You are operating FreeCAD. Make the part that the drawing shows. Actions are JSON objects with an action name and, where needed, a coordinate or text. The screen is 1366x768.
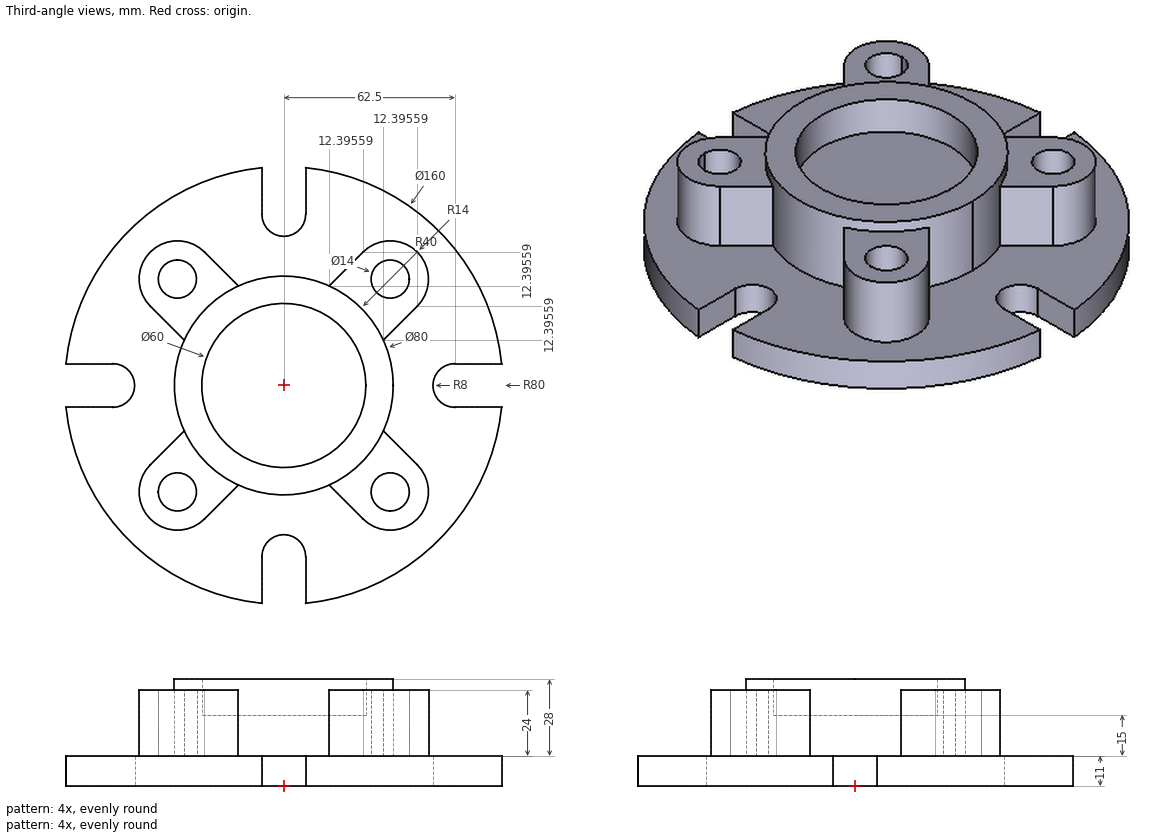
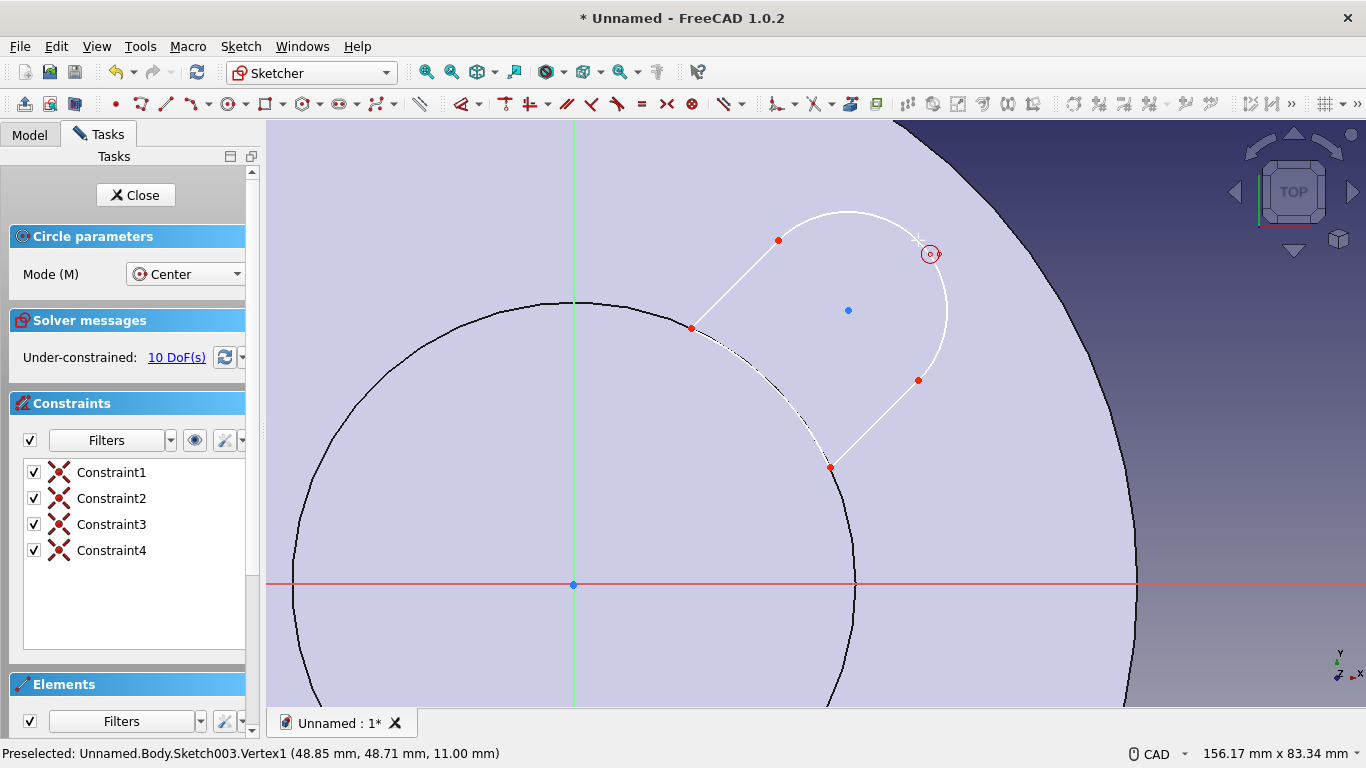
{"action": "left_click", "coordinate": [848, 310]}
{"action": "left_click", "coordinate": [883, 275]}
{"action": "key", "text": "Escape"}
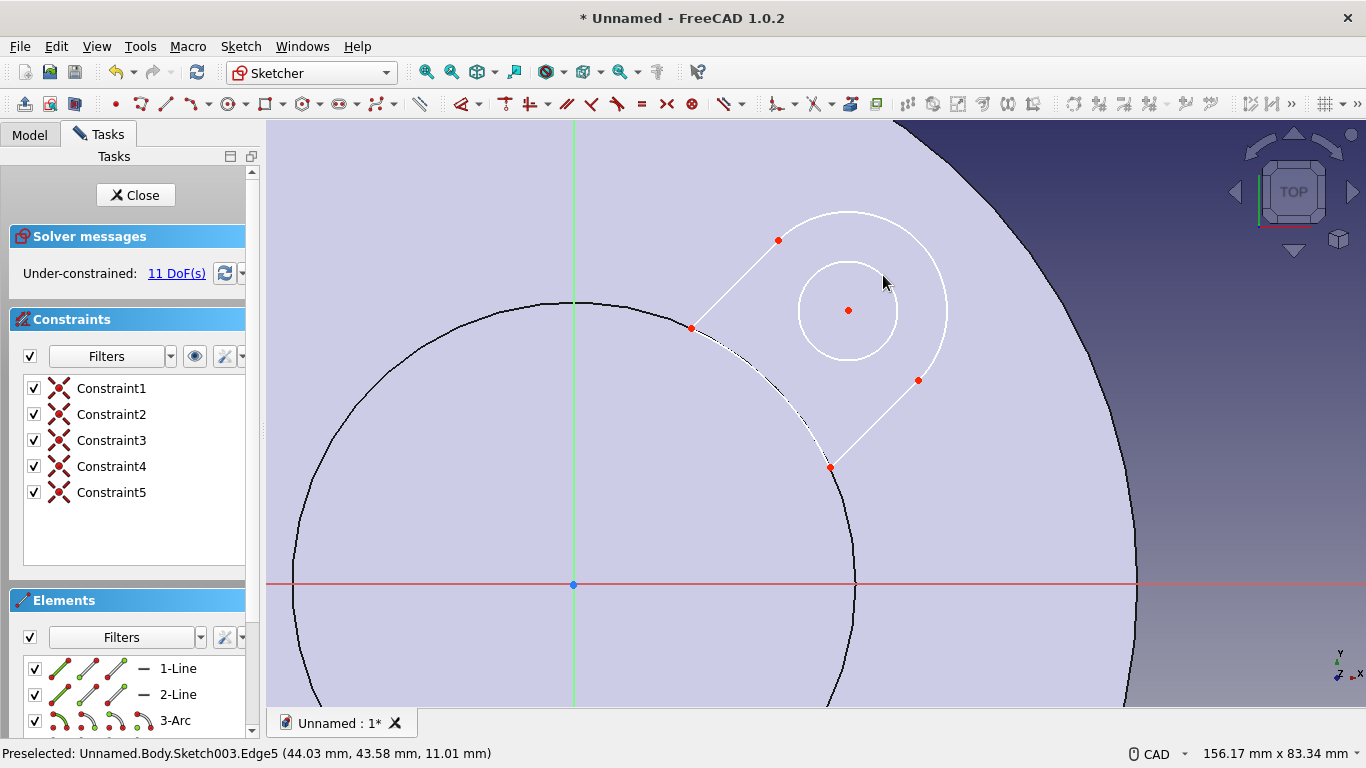
{"action": "left_click", "coordinate": [752, 267]}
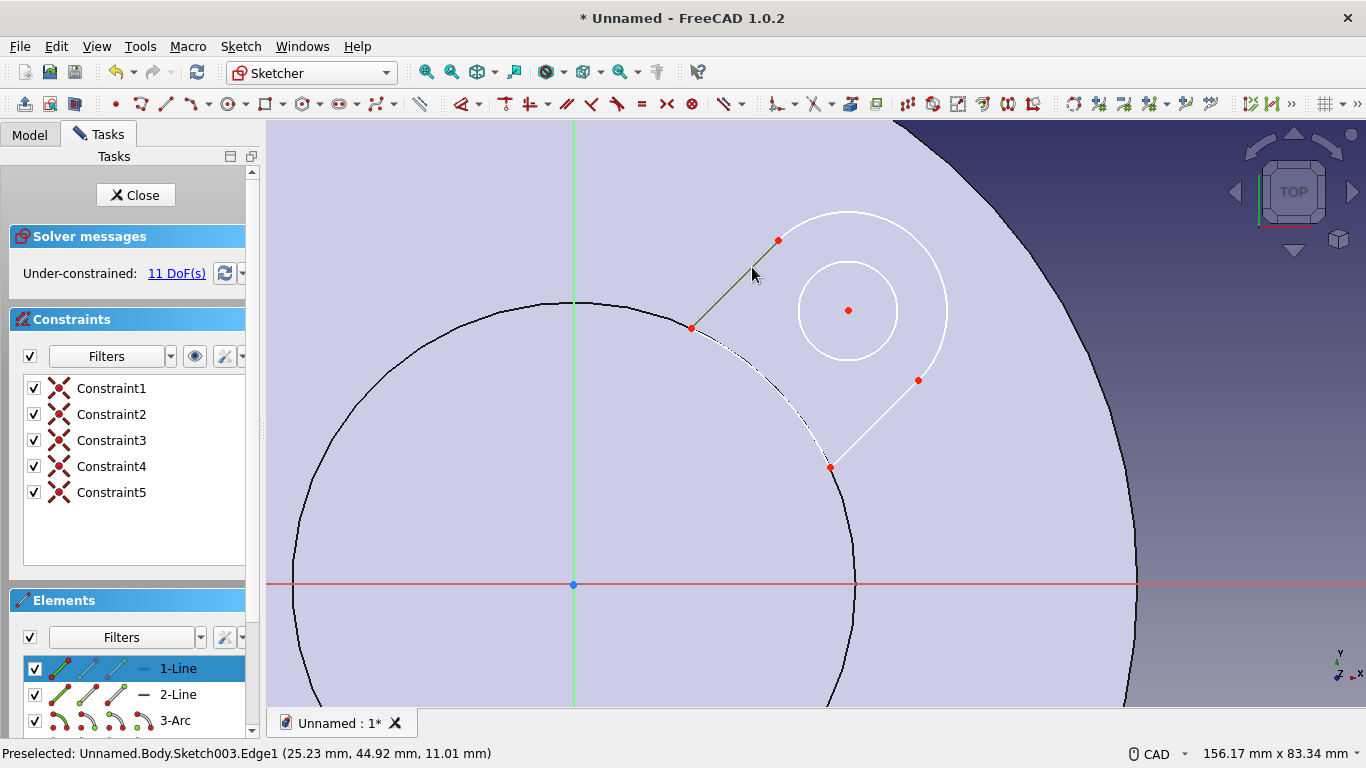
{"action": "left_click", "coordinate": [946, 296]}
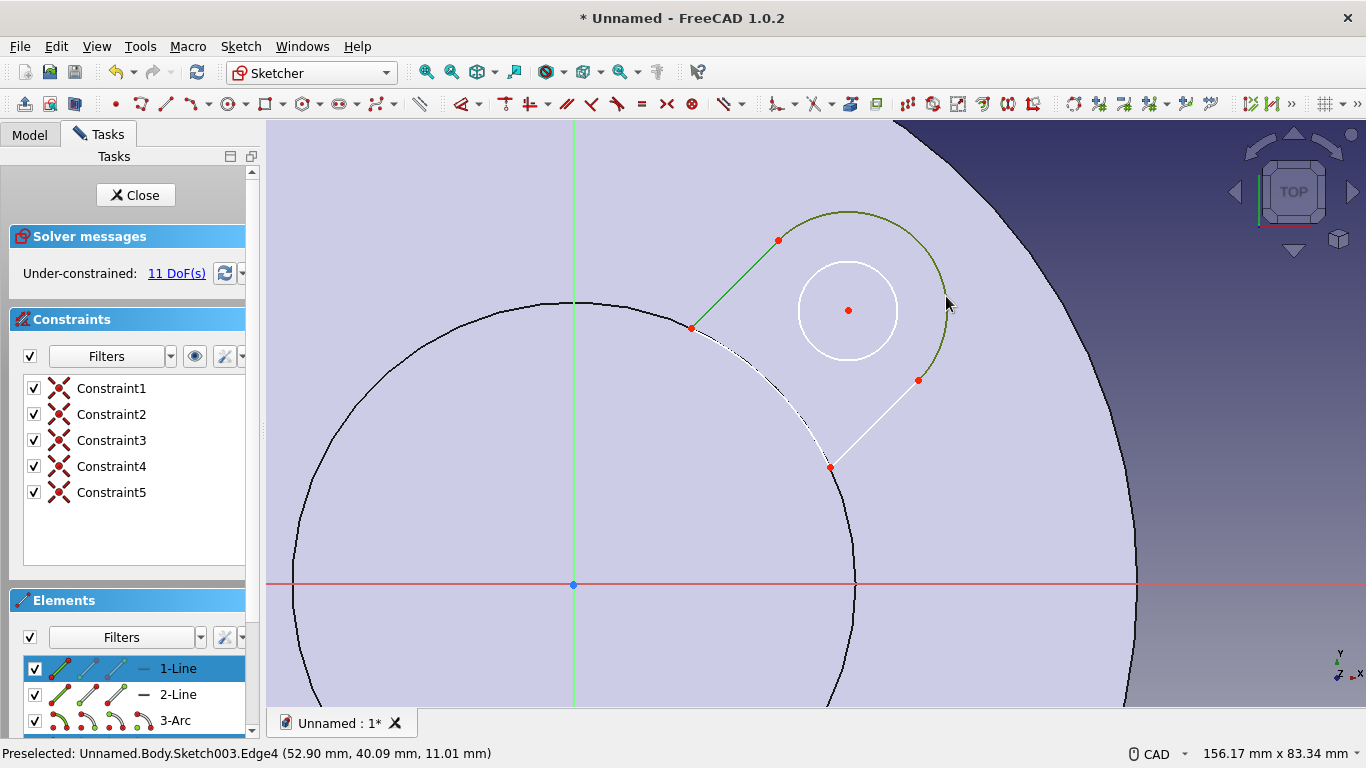
{"action": "key", "text": "t"}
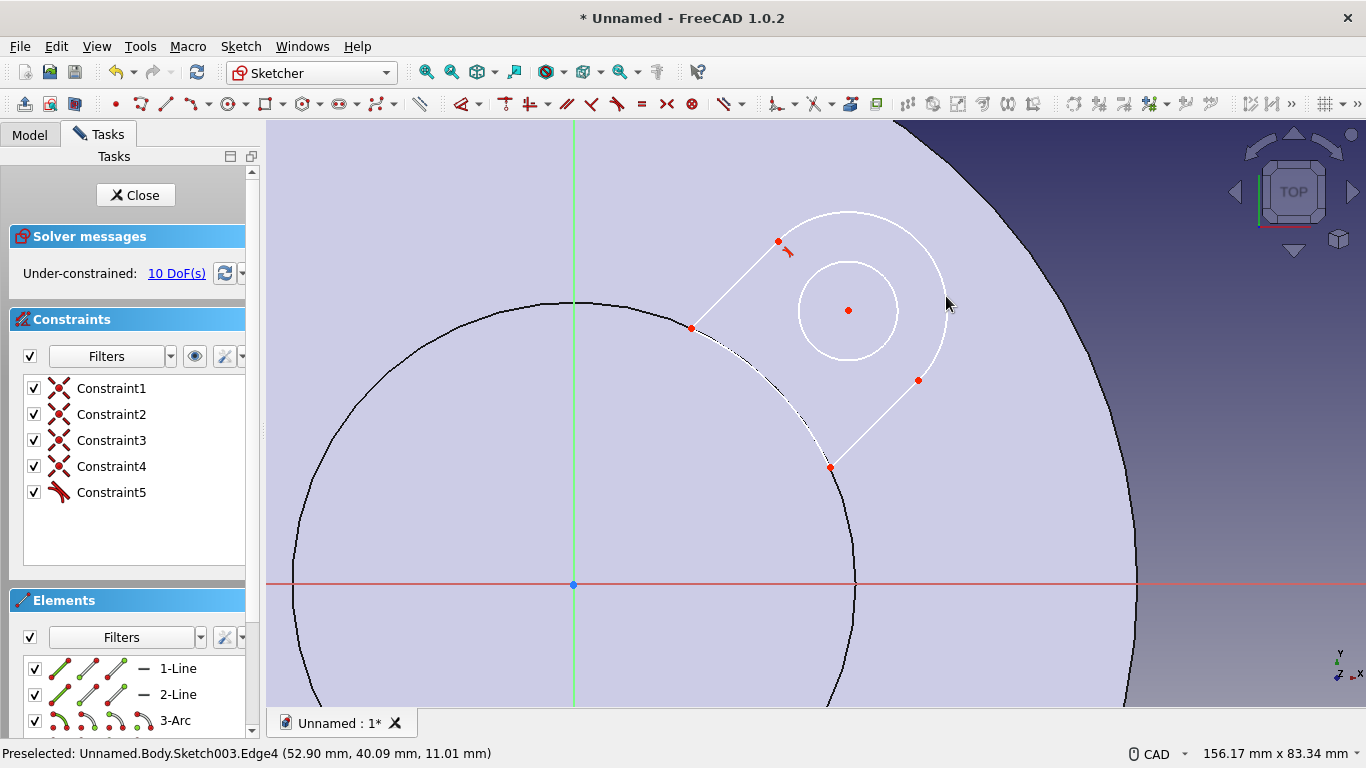
{"action": "left_click", "coordinate": [856, 442]}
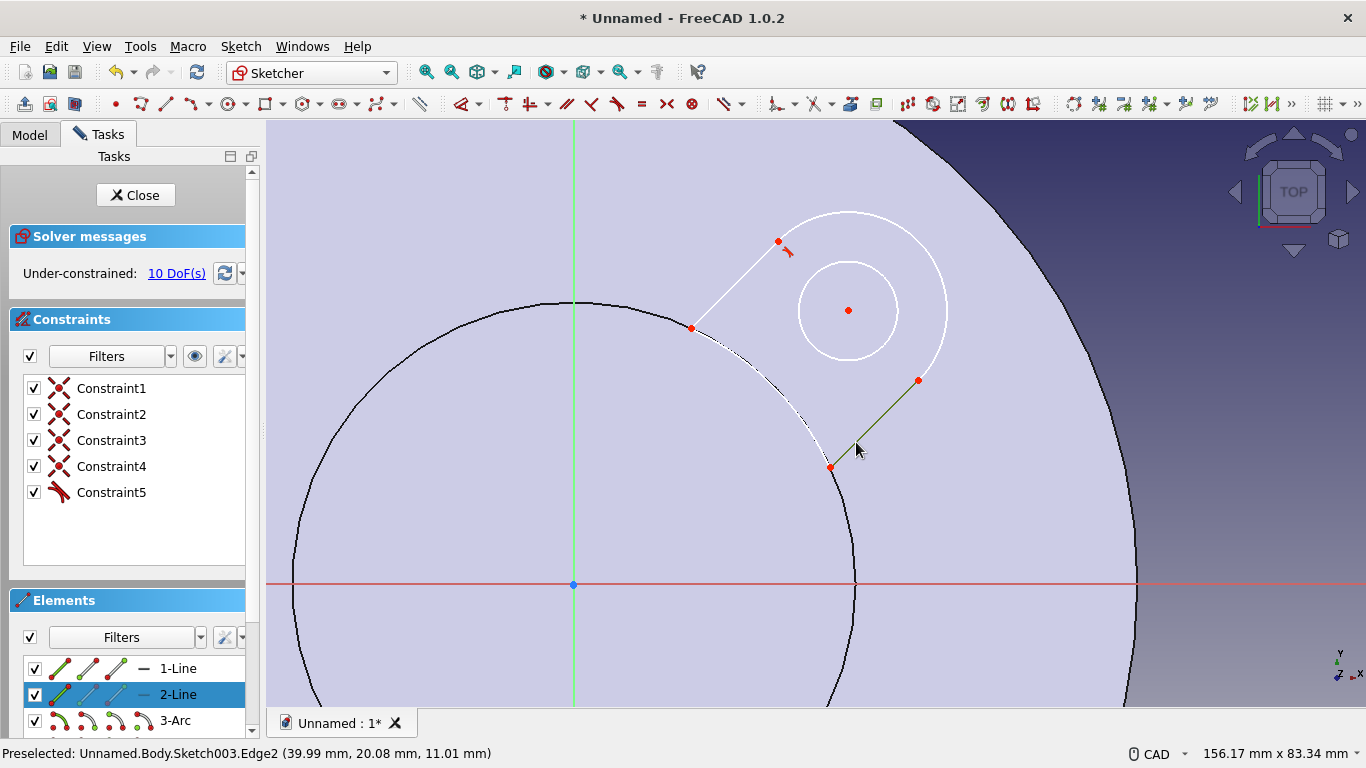
{"action": "left_click", "coordinate": [946, 296]}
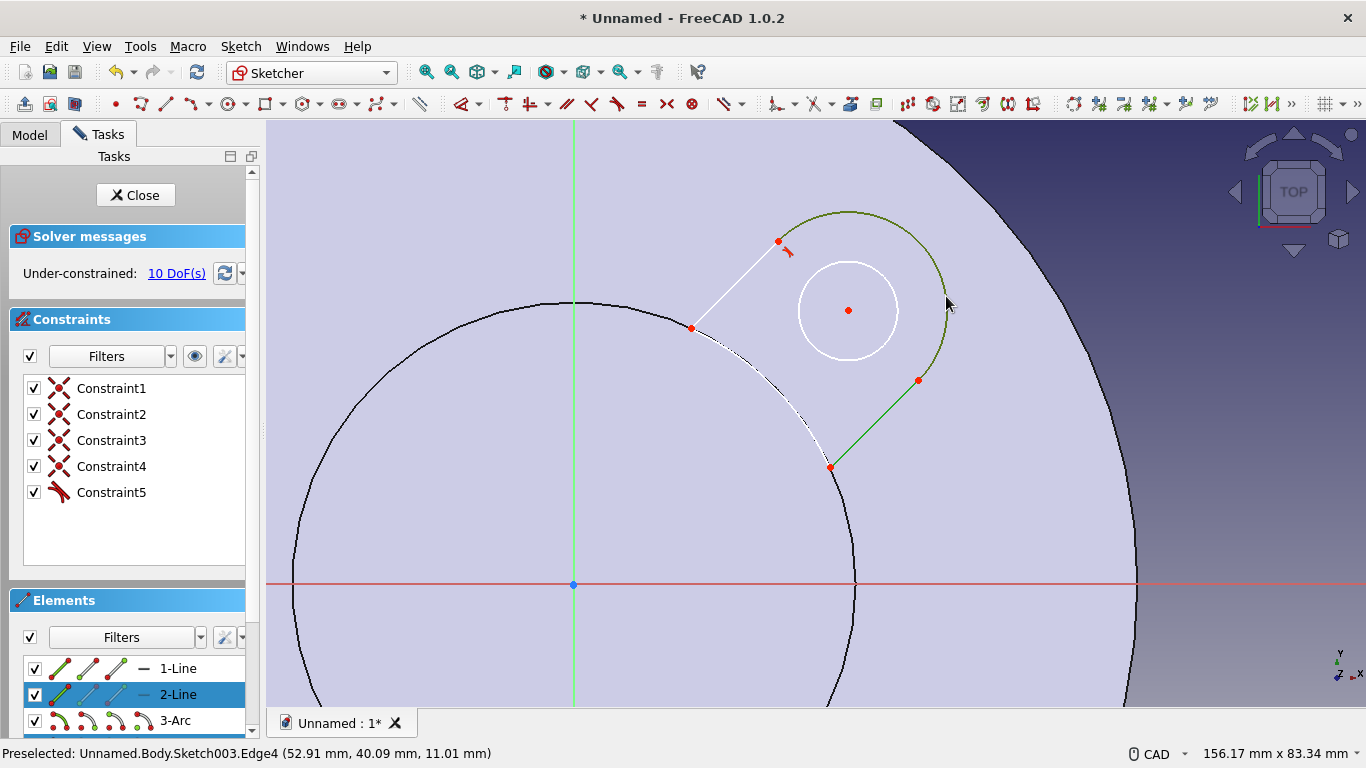
{"action": "key", "text": "t"}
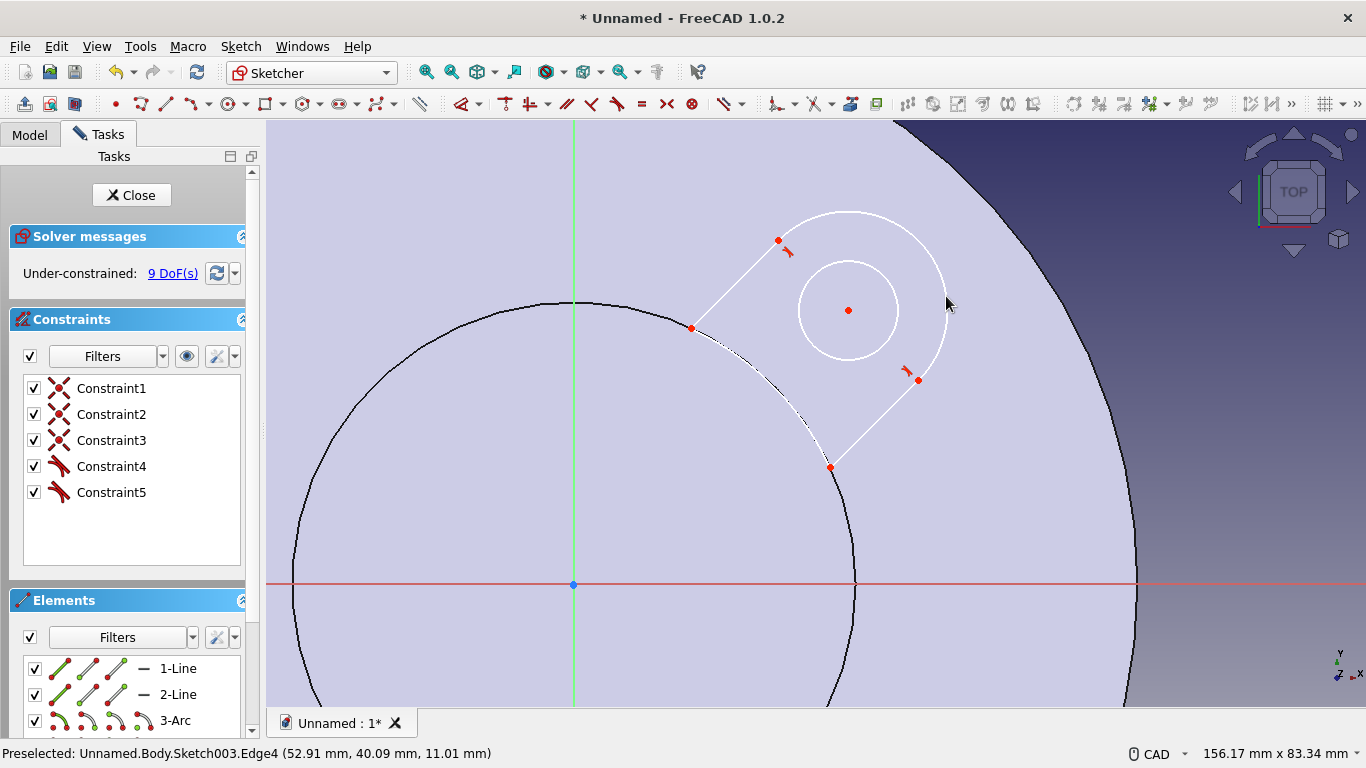
{"action": "left_click_drag", "start_coordinate": [564, 574], "coordinate": [584, 595]}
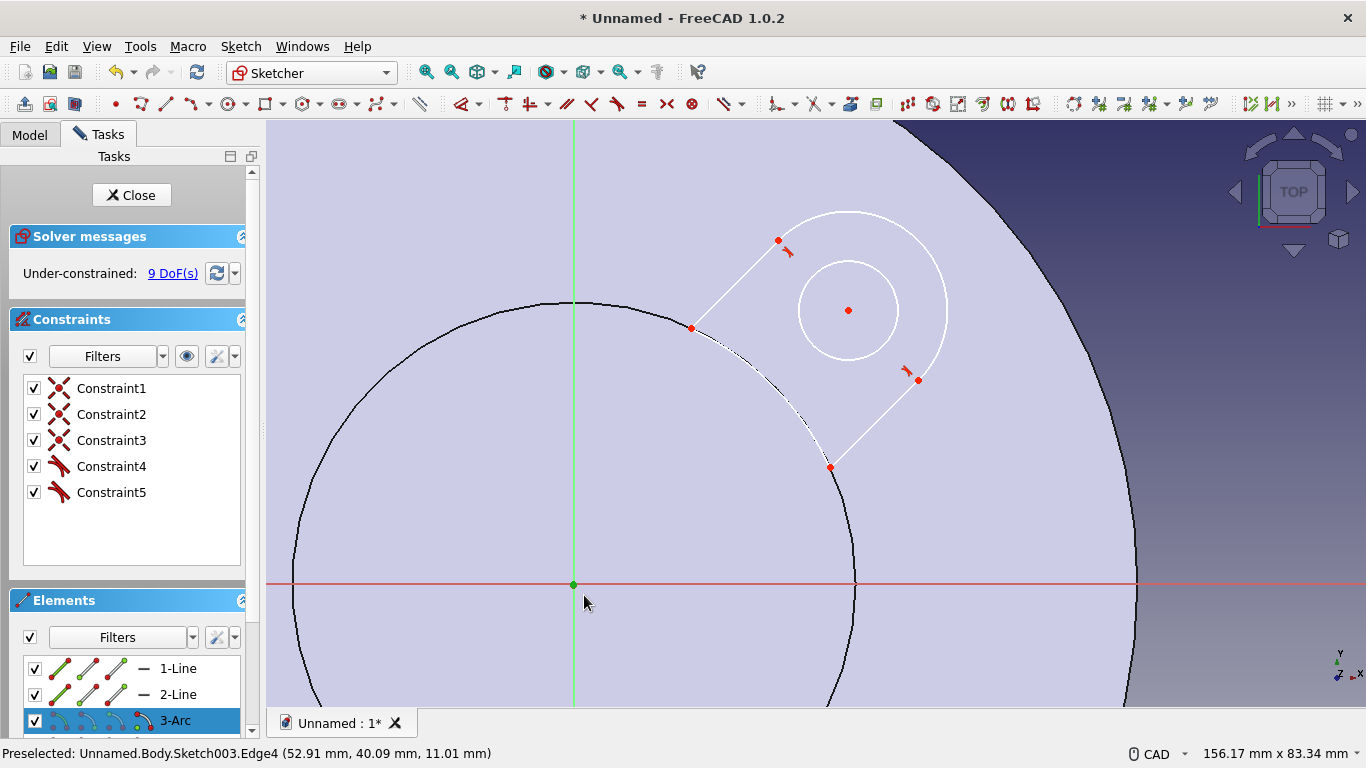
{"action": "key", "text": "c"}